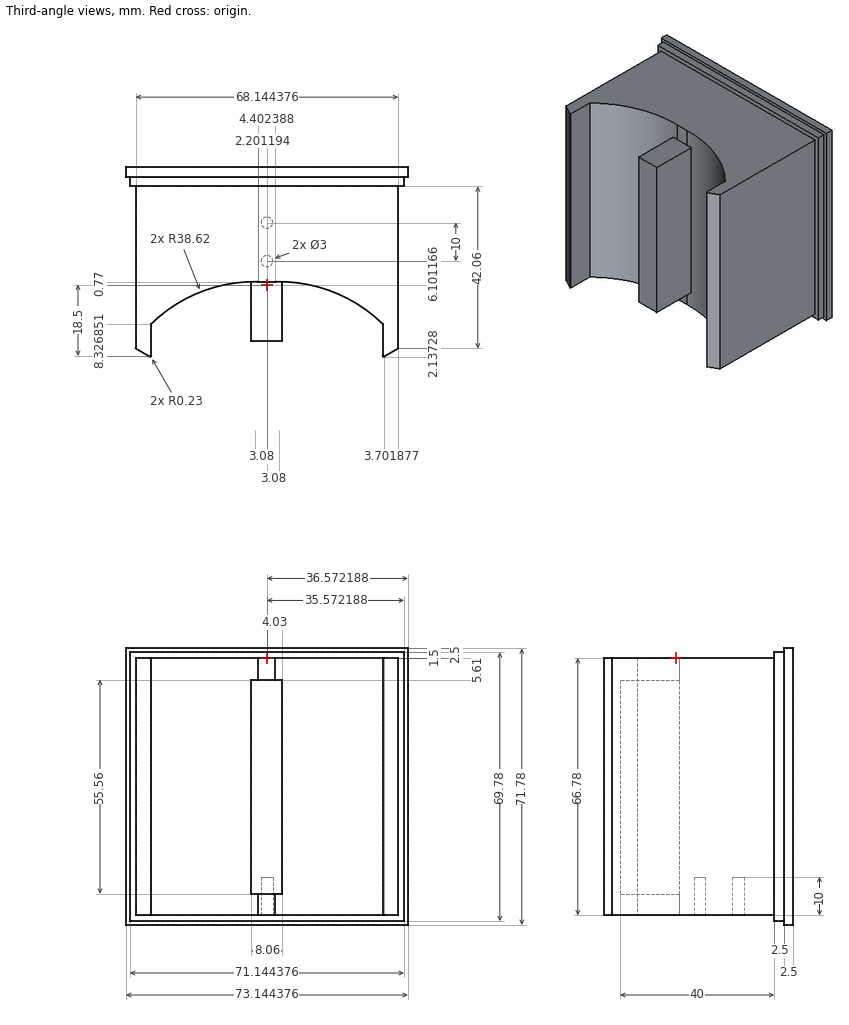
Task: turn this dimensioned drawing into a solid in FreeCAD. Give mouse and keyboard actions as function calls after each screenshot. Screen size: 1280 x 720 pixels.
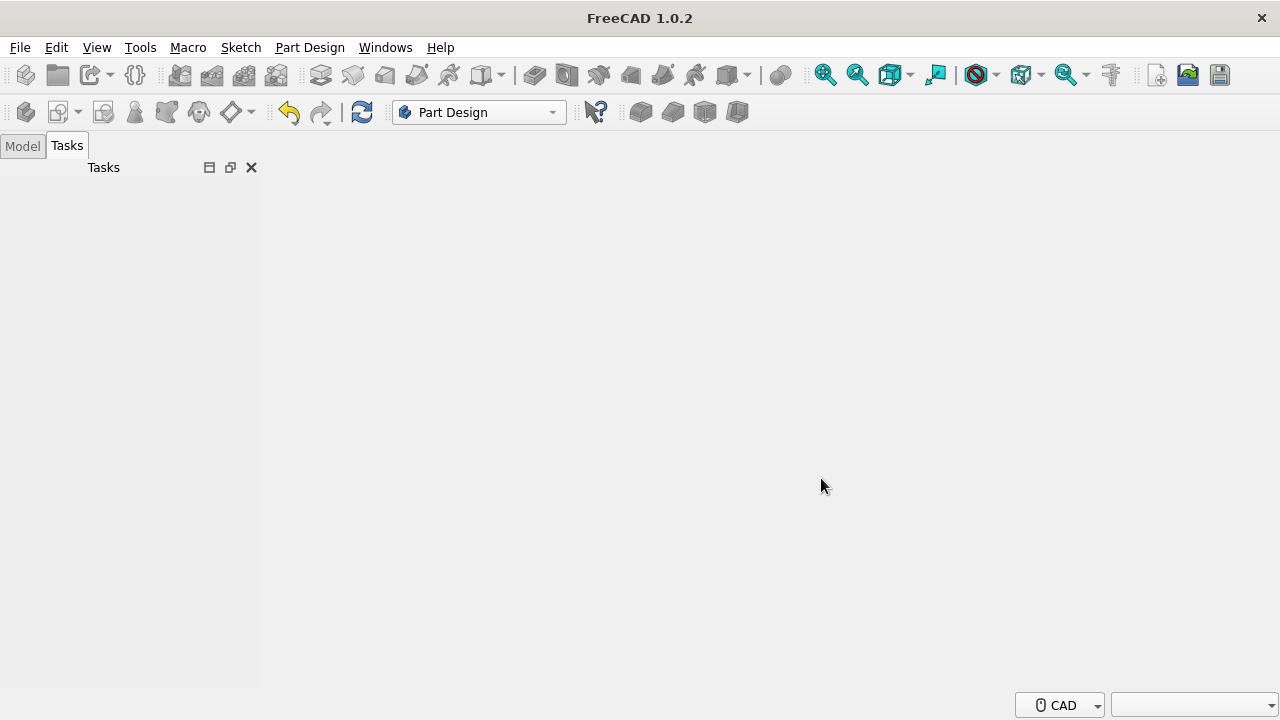
click(1156, 76)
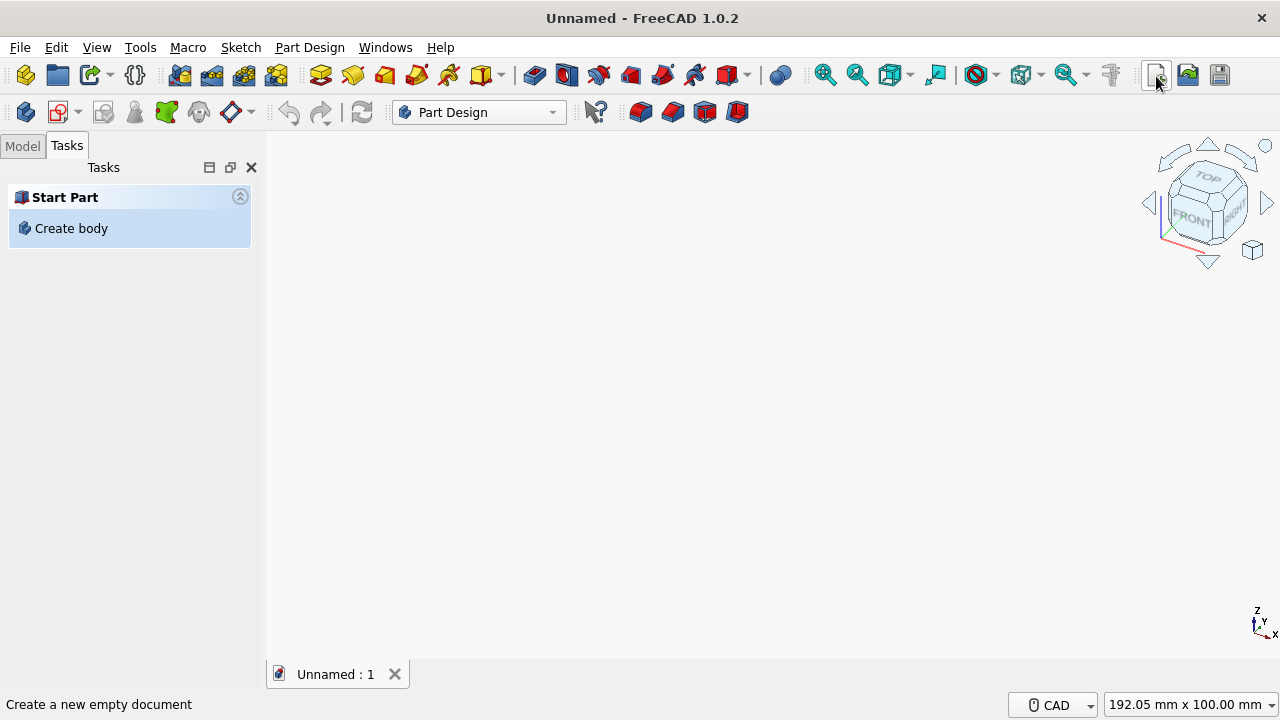
click(58, 112)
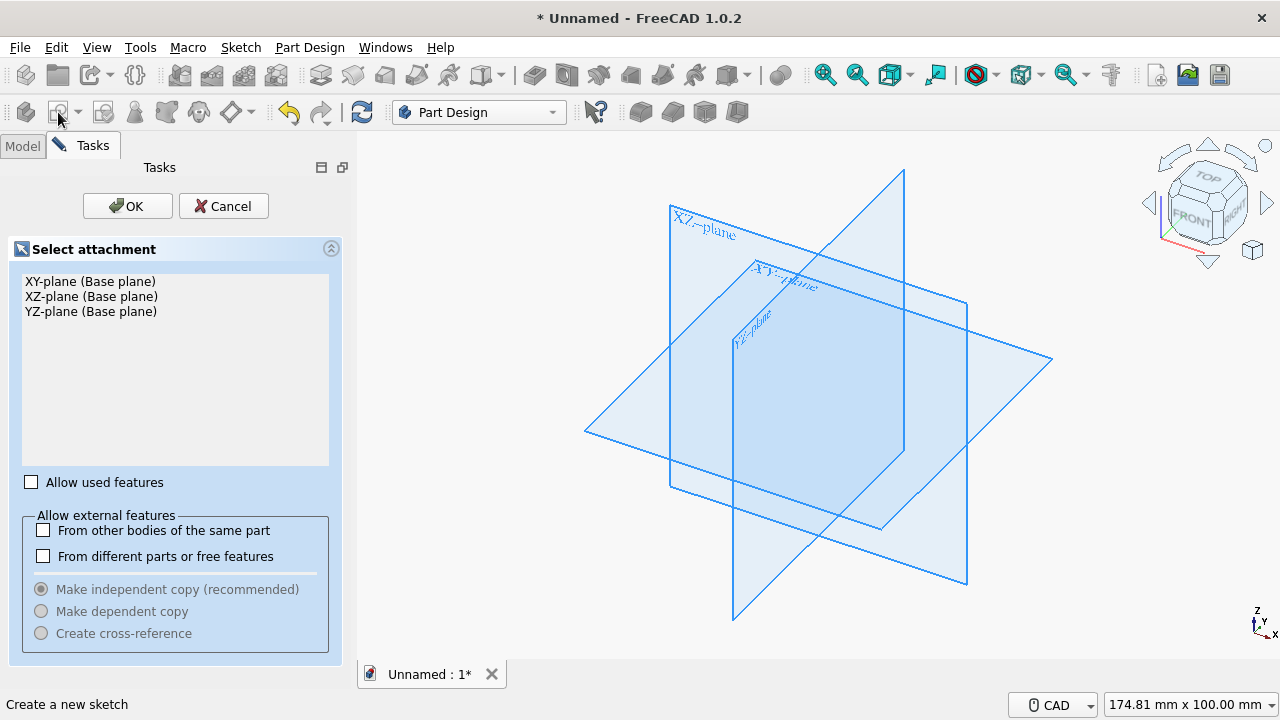
click(82, 282)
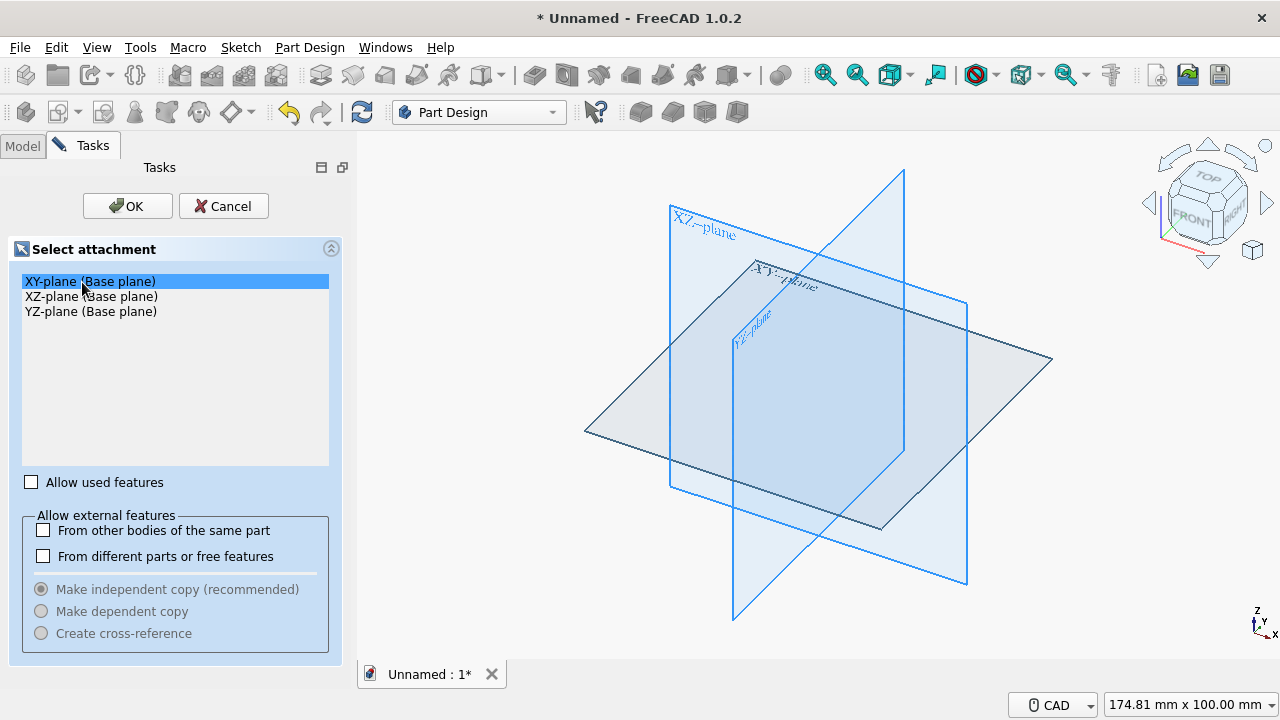
click(128, 206)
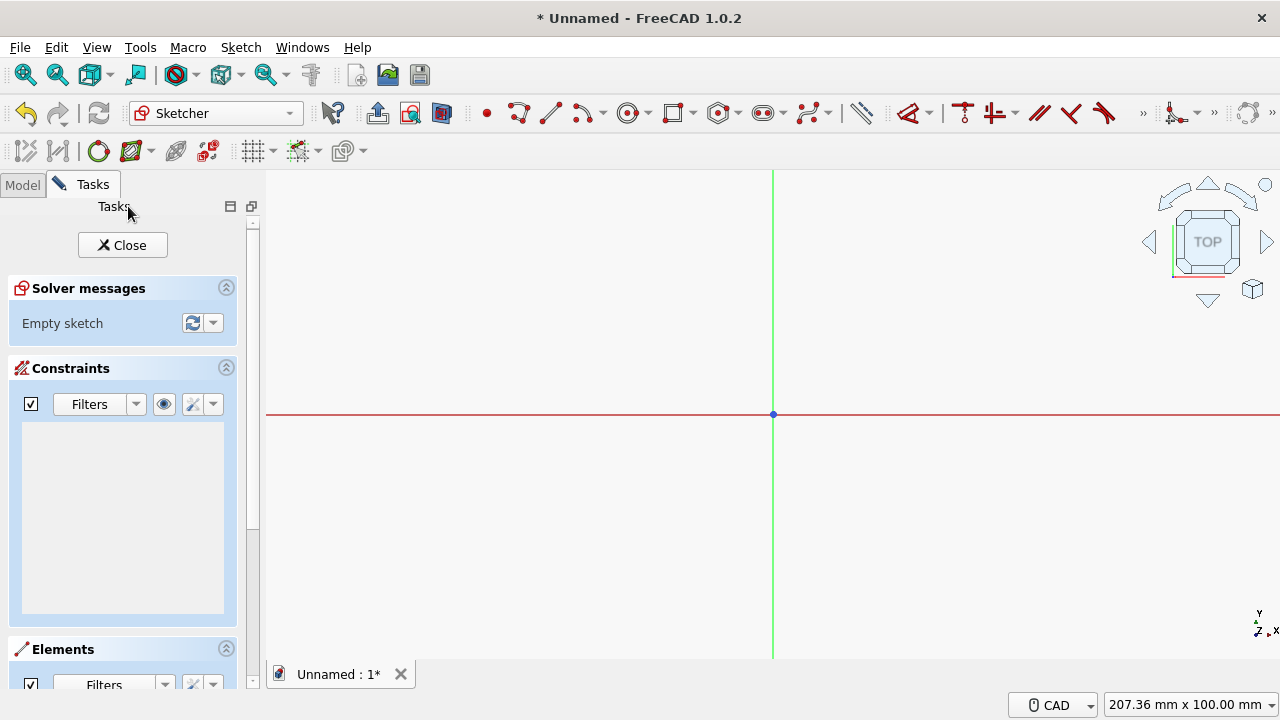
scroll(912, 364, up, 2)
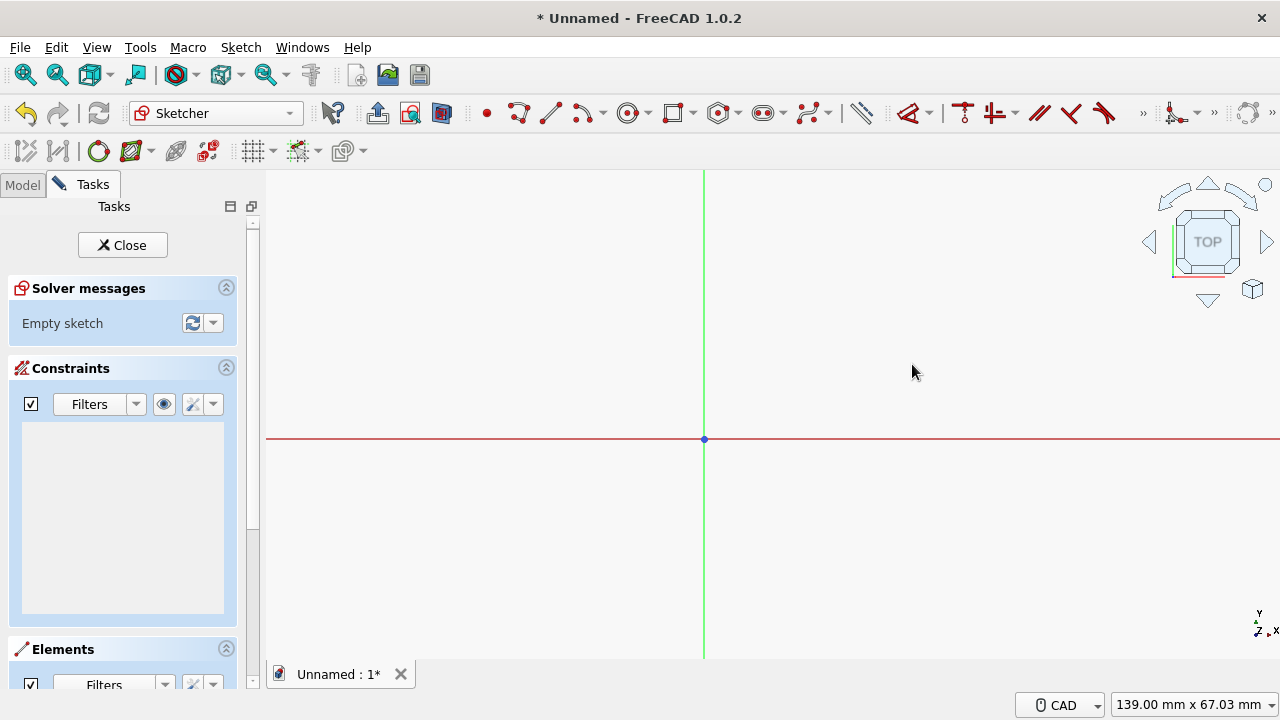
click(552, 114)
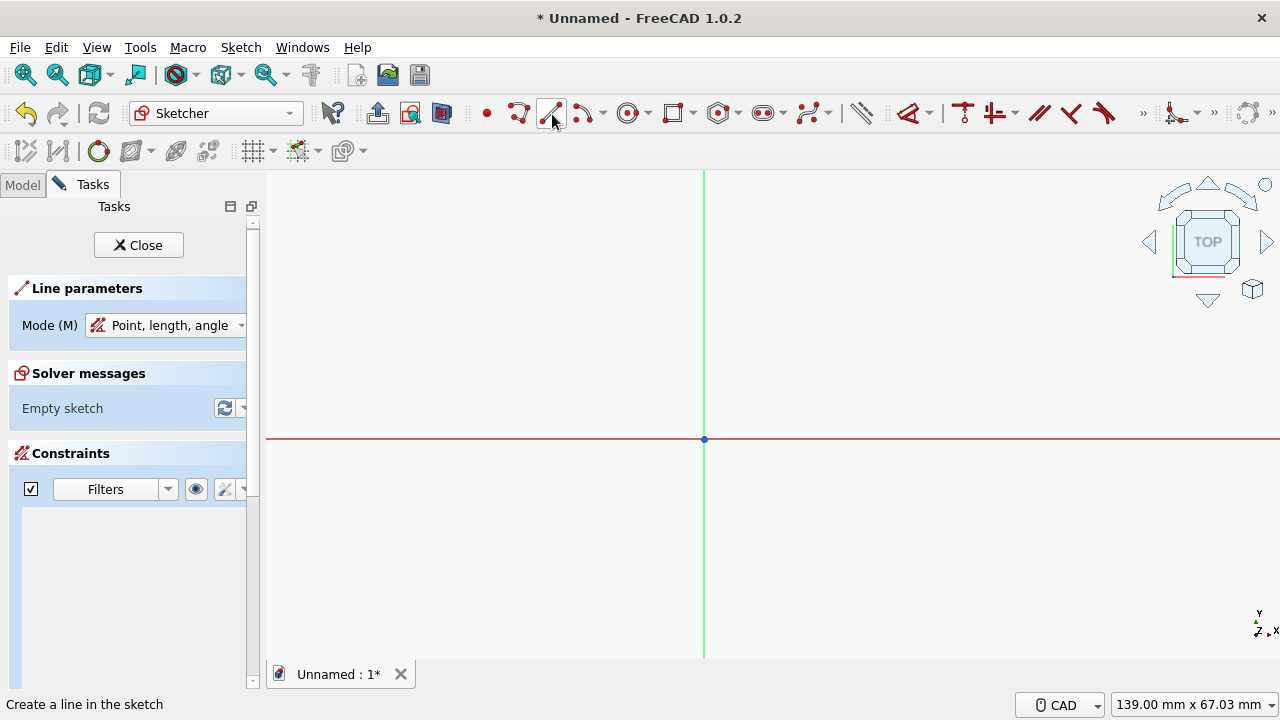
click(485, 574)
click(485, 513)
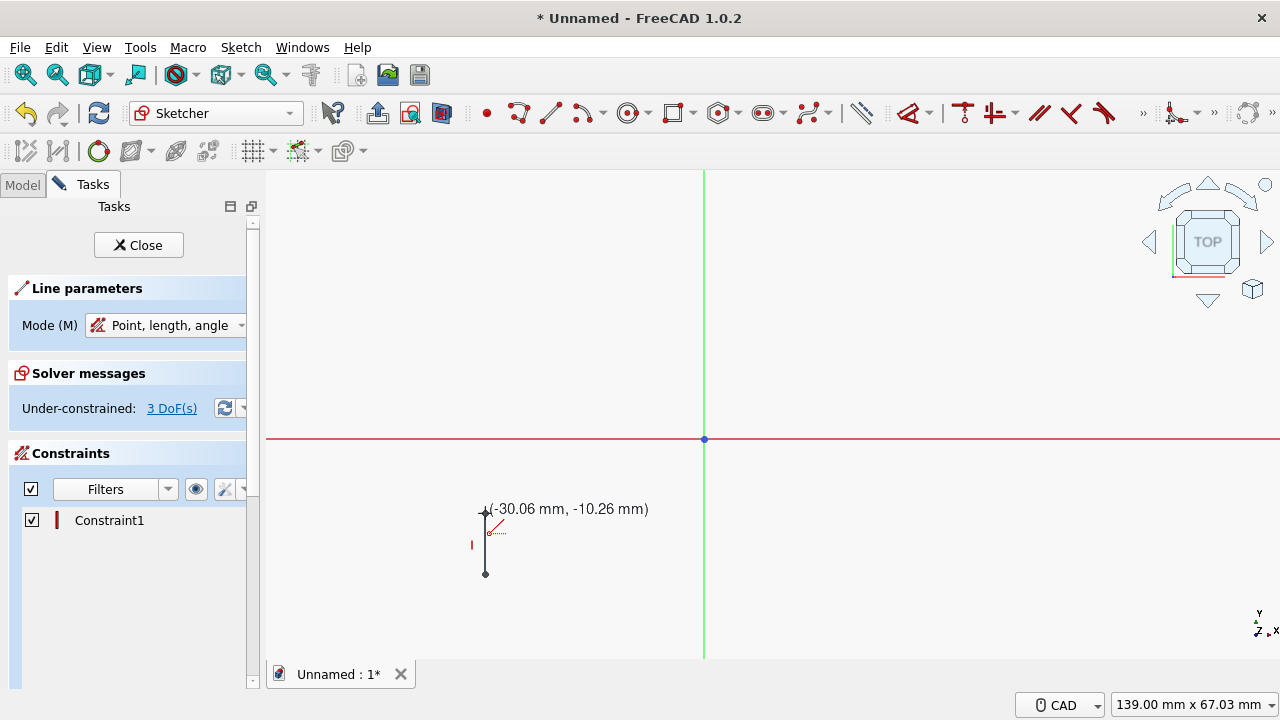
scroll(688, 434, up, 6)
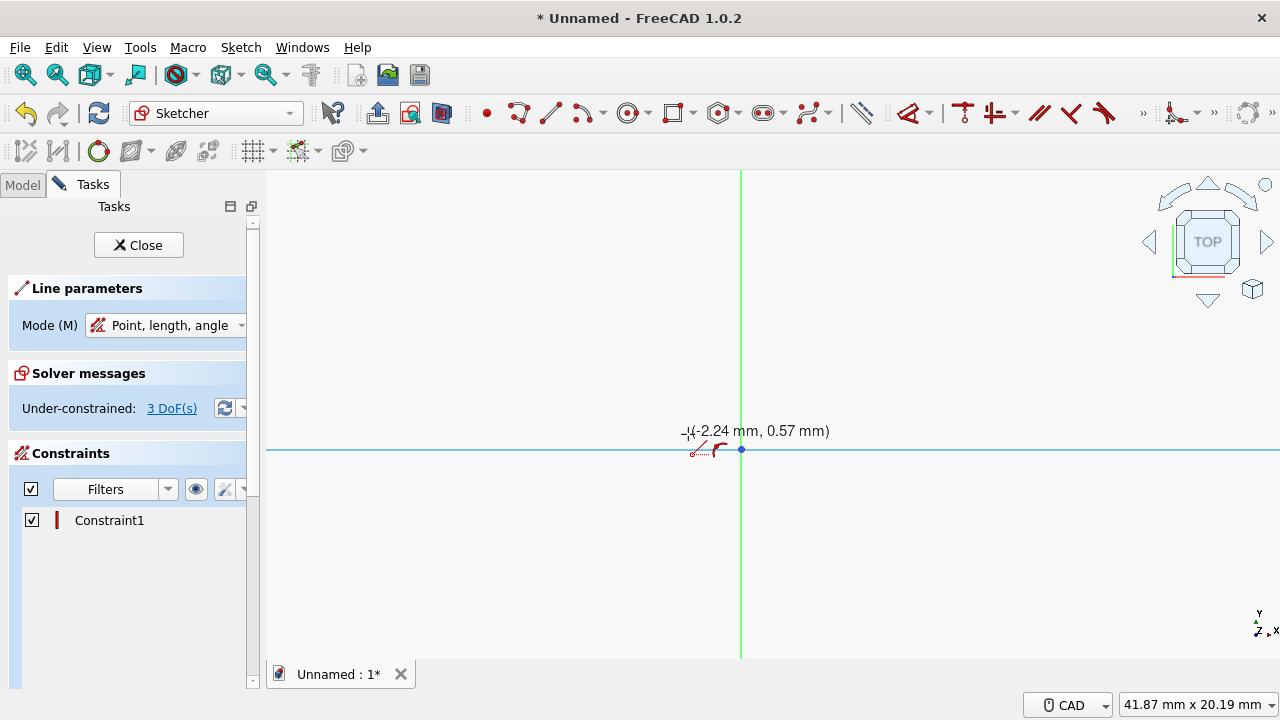
click(688, 431)
click(795, 431)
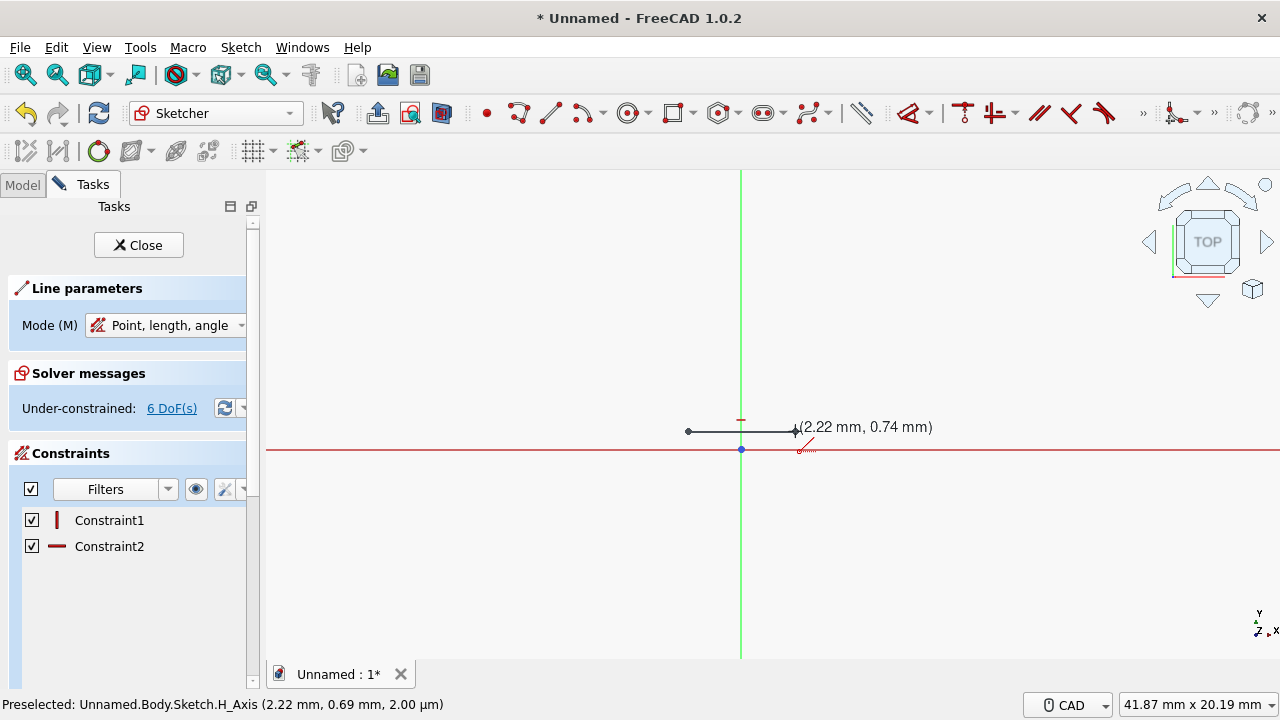
scroll(689, 435, down, 6)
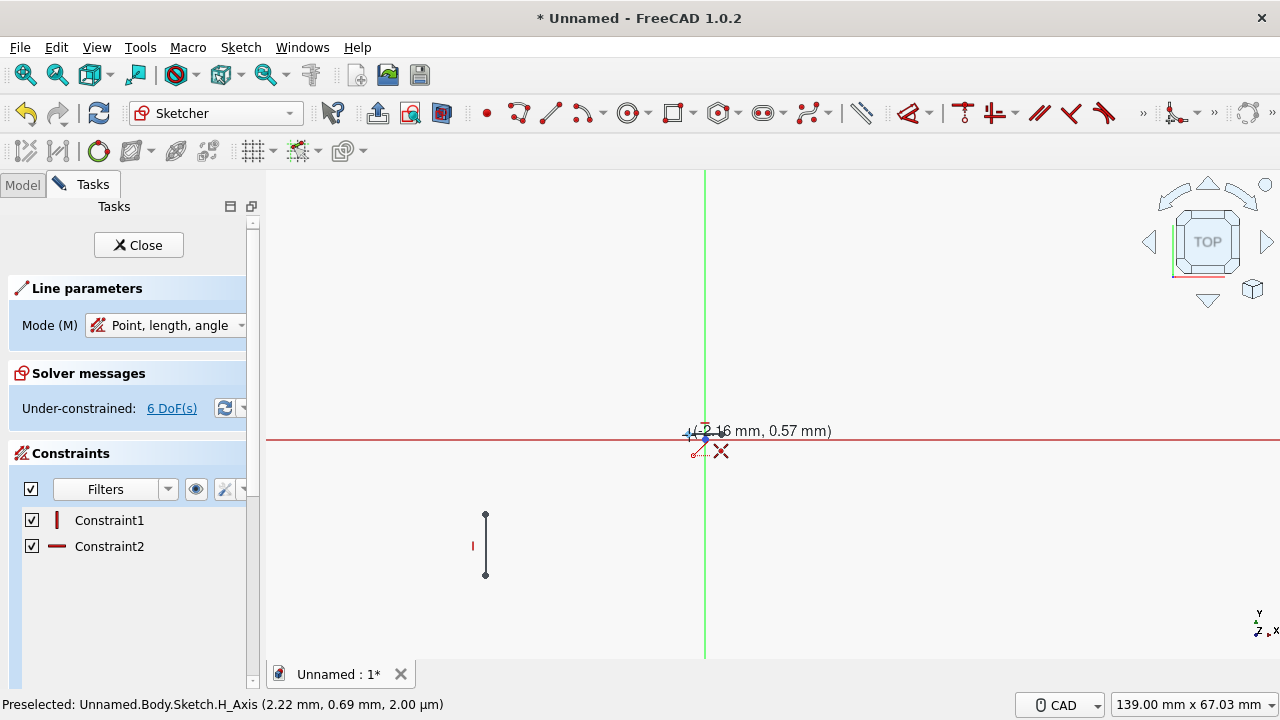
click(924, 514)
click(924, 575)